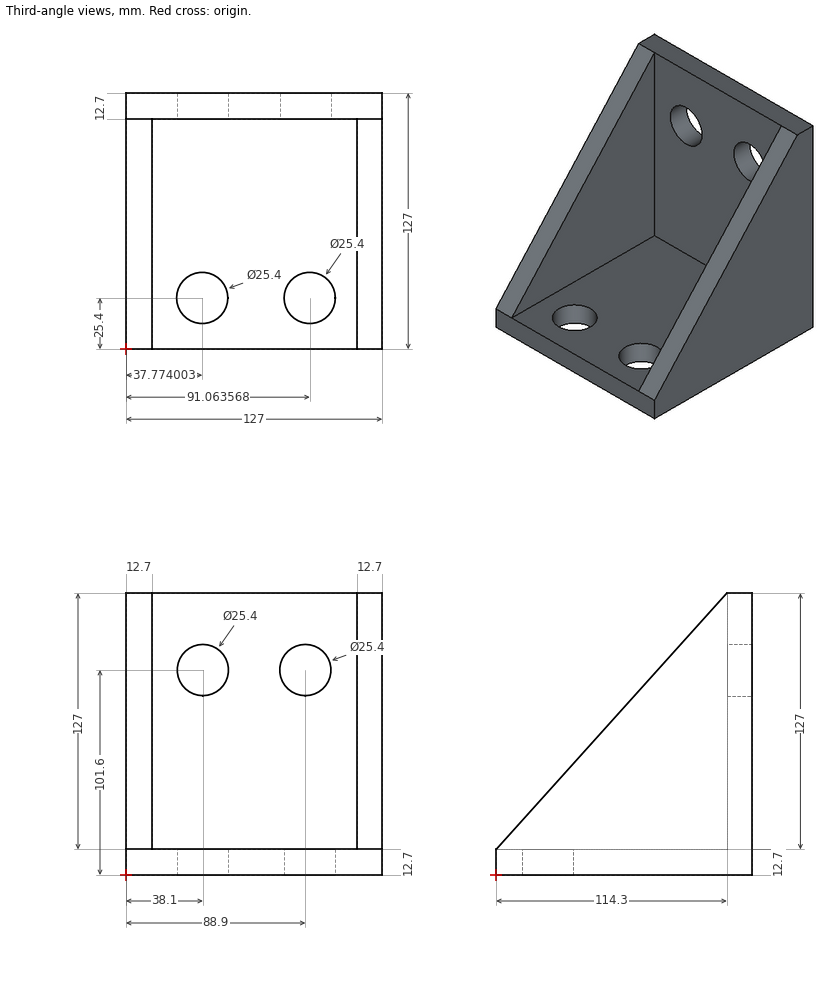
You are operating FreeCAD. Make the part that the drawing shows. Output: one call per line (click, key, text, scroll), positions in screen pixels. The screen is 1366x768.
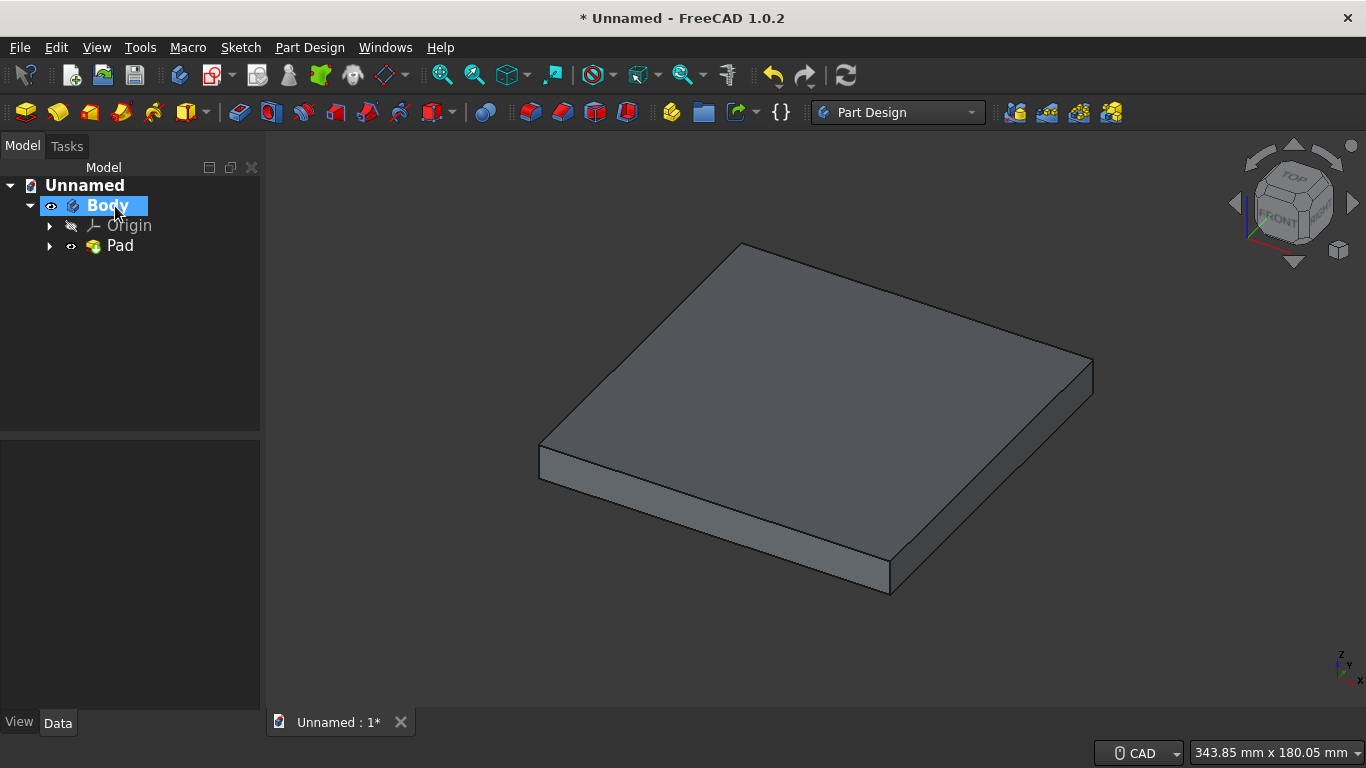
click(816, 401)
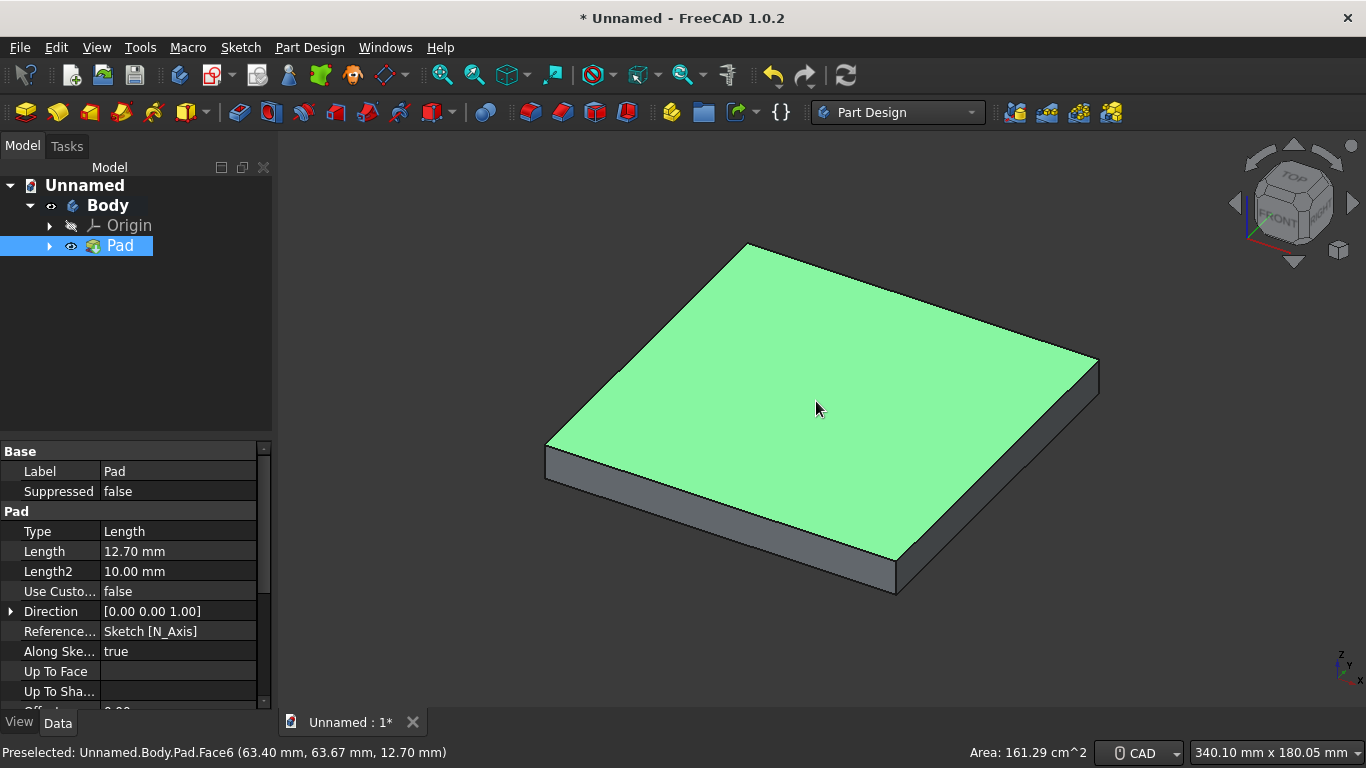
click(212, 76)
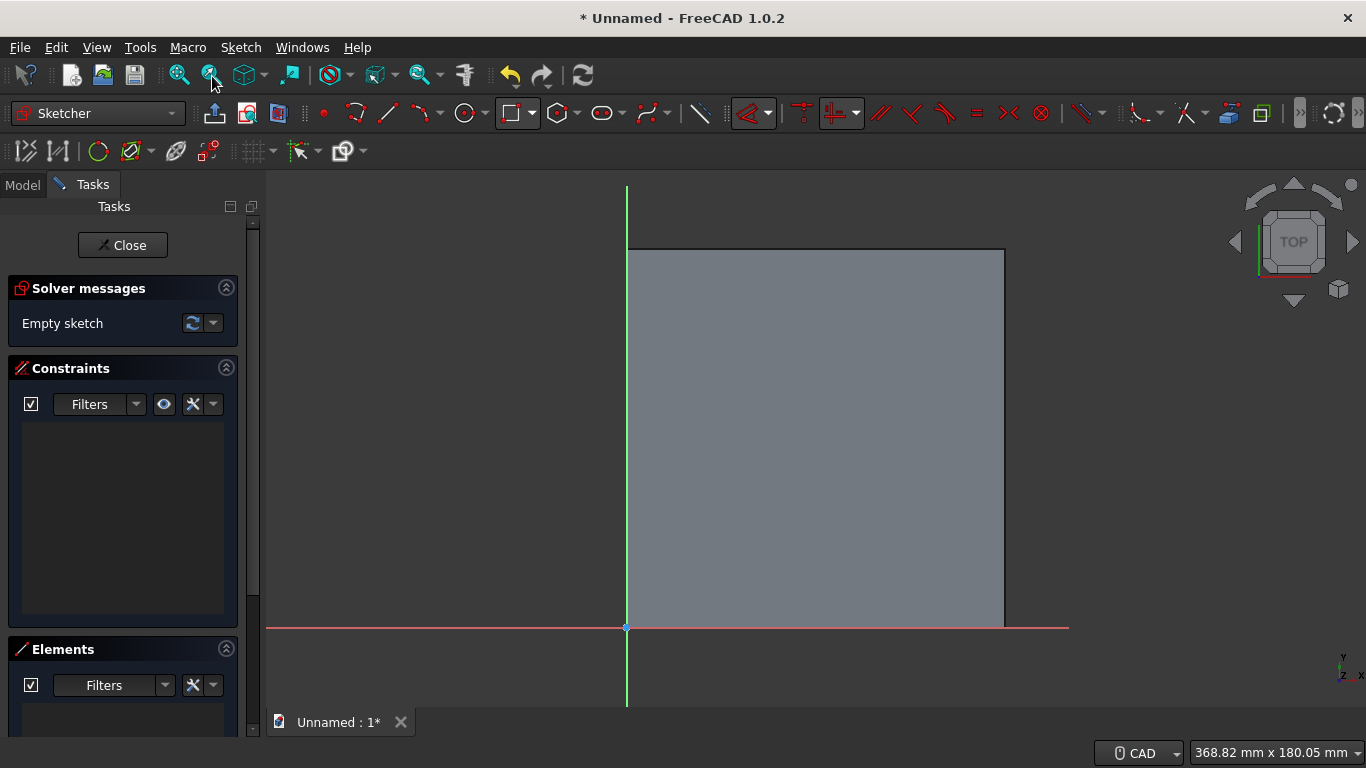
key(g)
key(r)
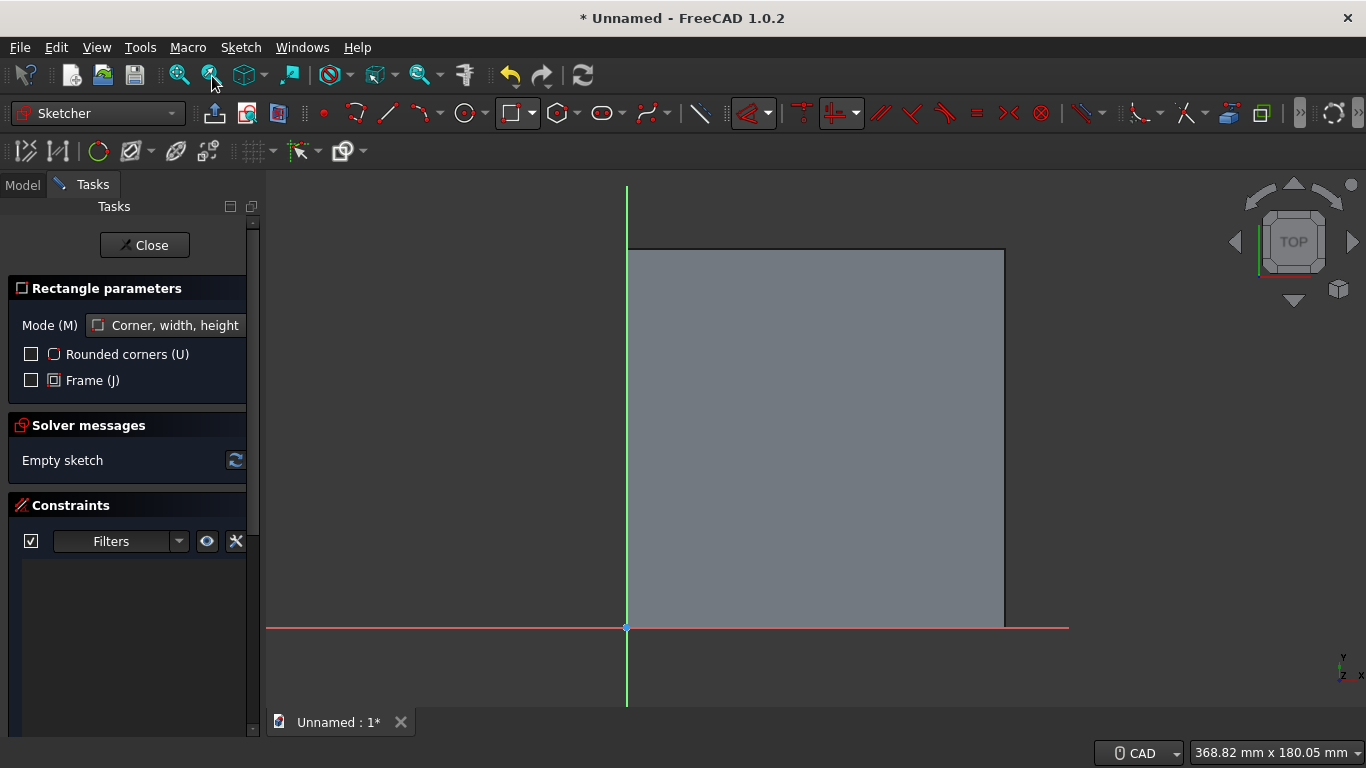
click(627, 249)
click(1005, 287)
key(Escape)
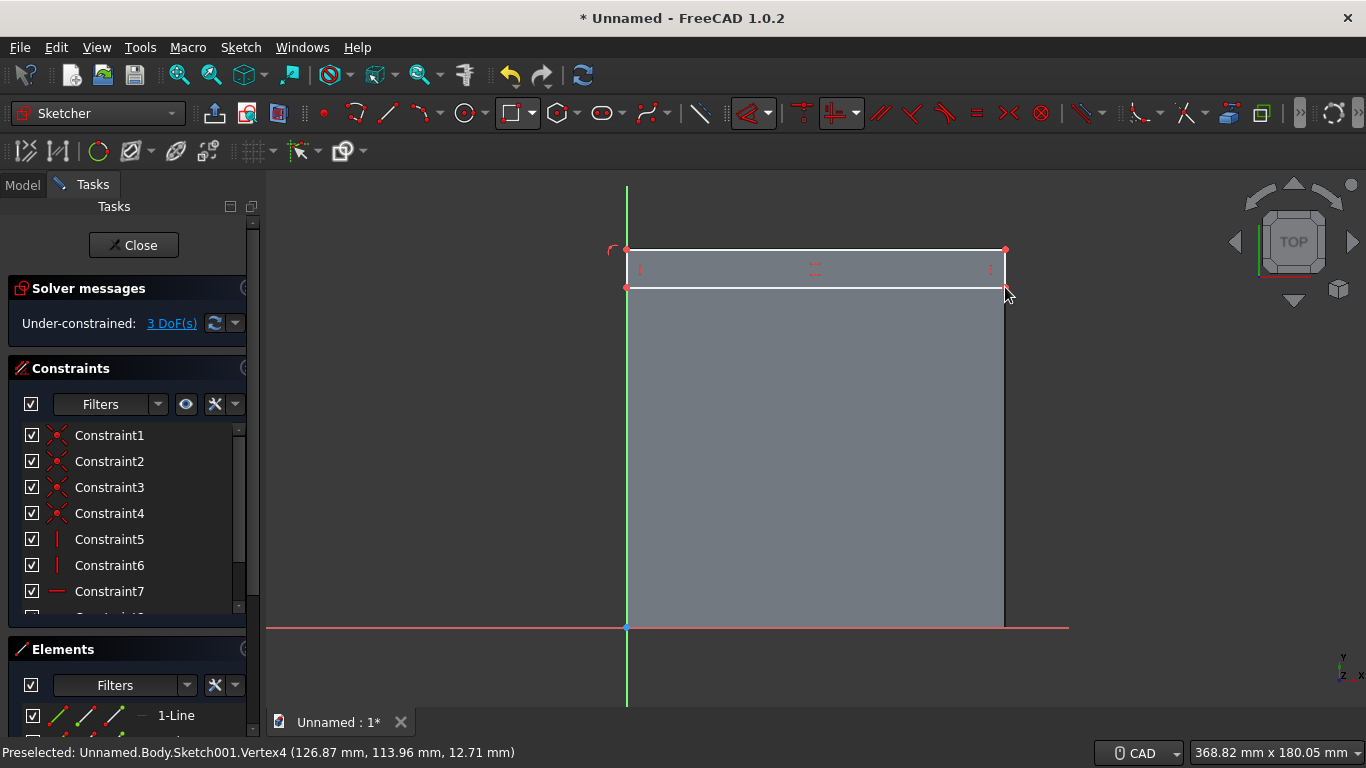
click(740, 288)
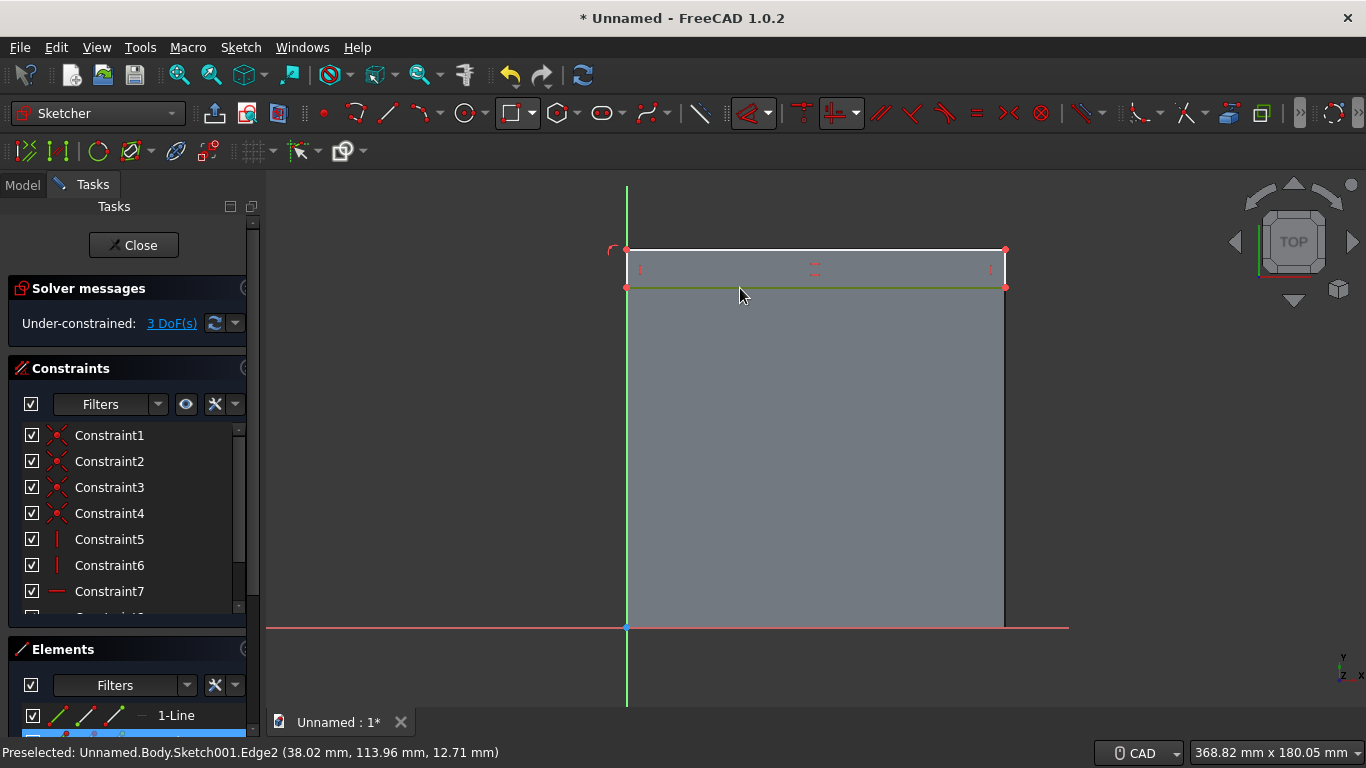
key(l)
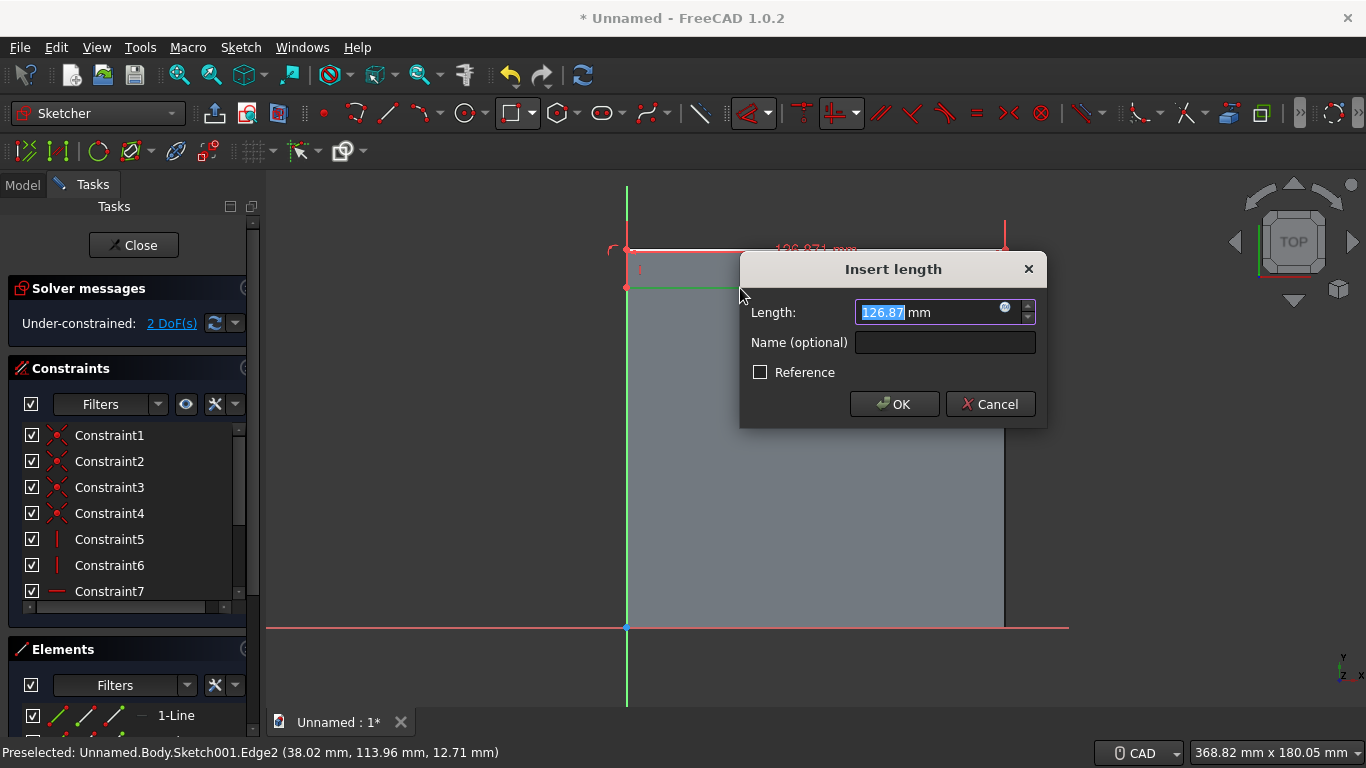
text(127)
key(Return)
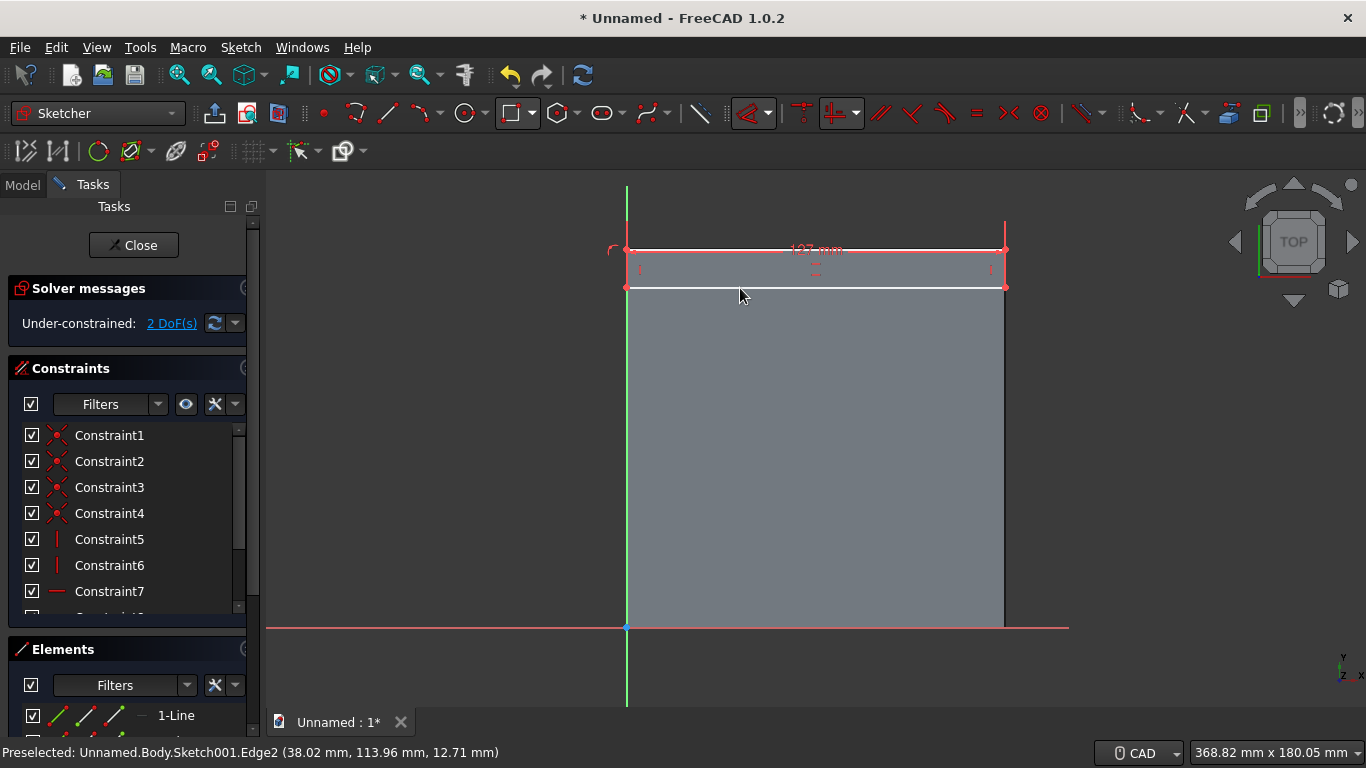
click(627, 261)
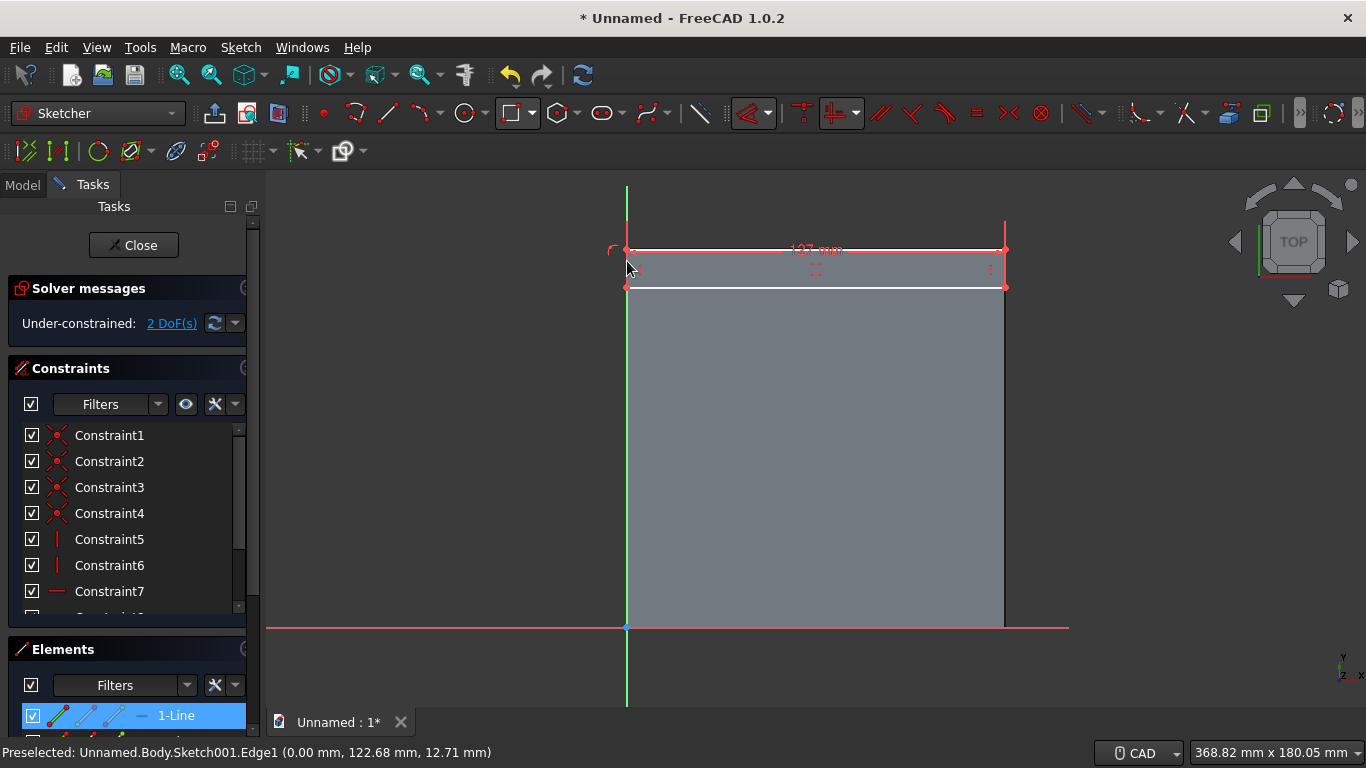
key(i)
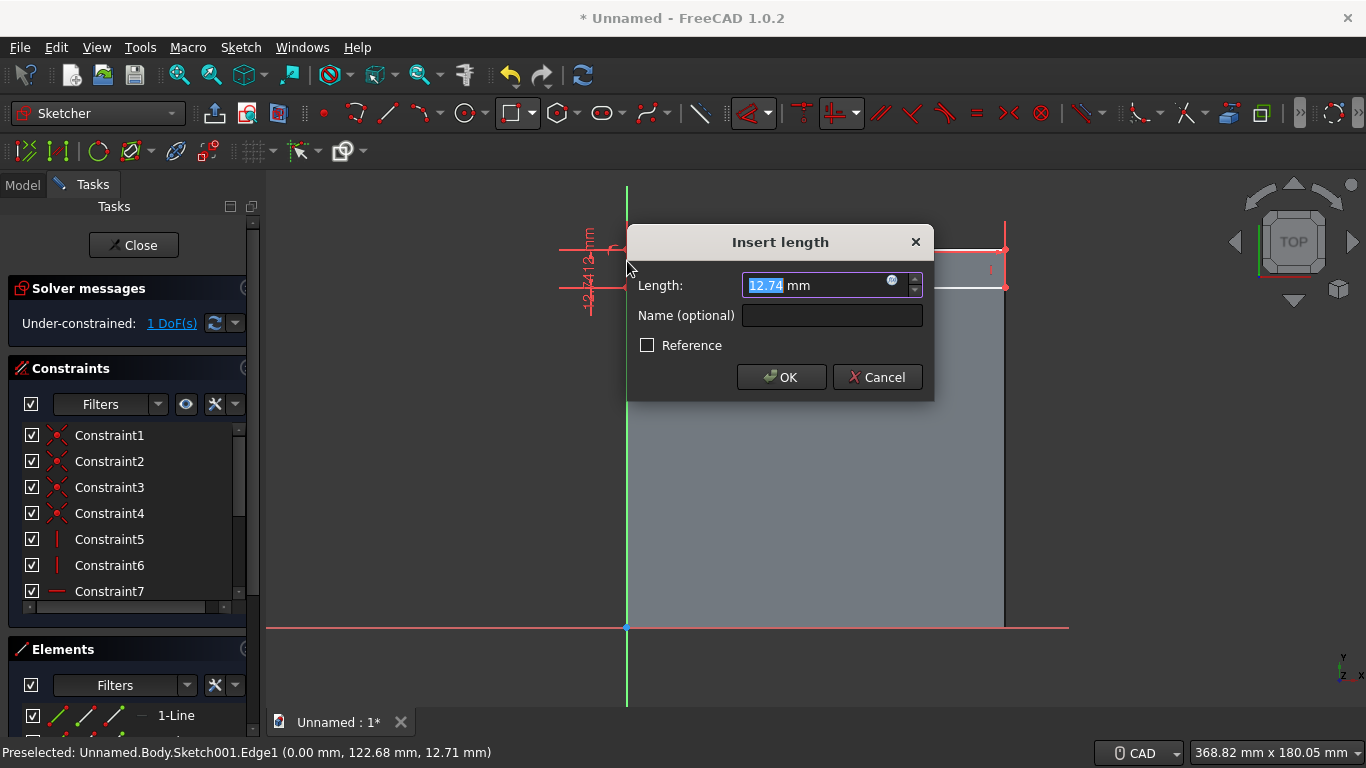
text(12.7)
key(Return)